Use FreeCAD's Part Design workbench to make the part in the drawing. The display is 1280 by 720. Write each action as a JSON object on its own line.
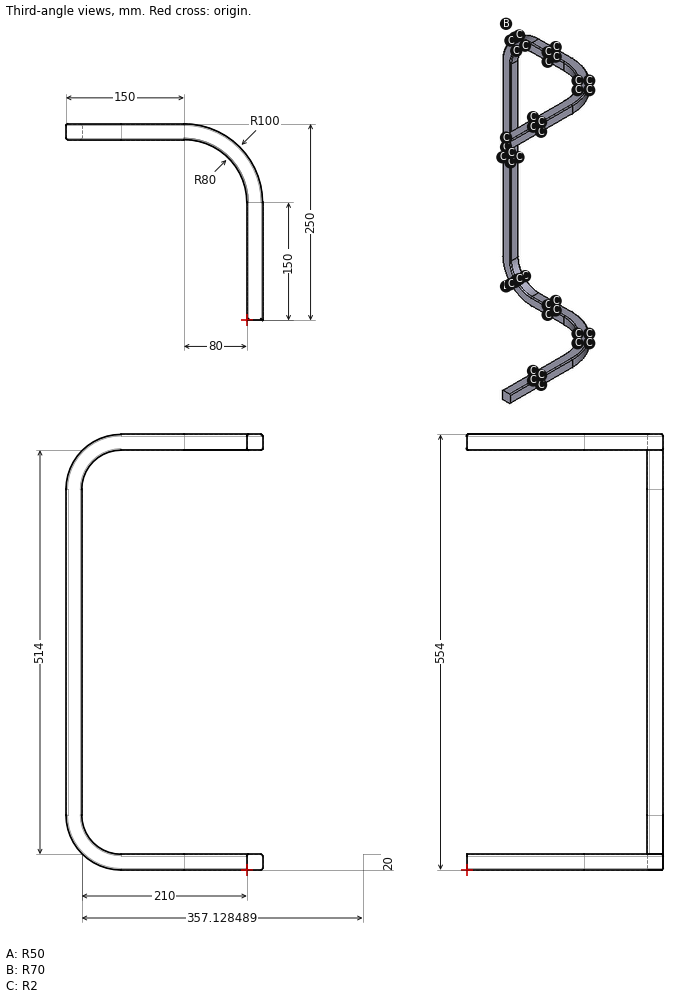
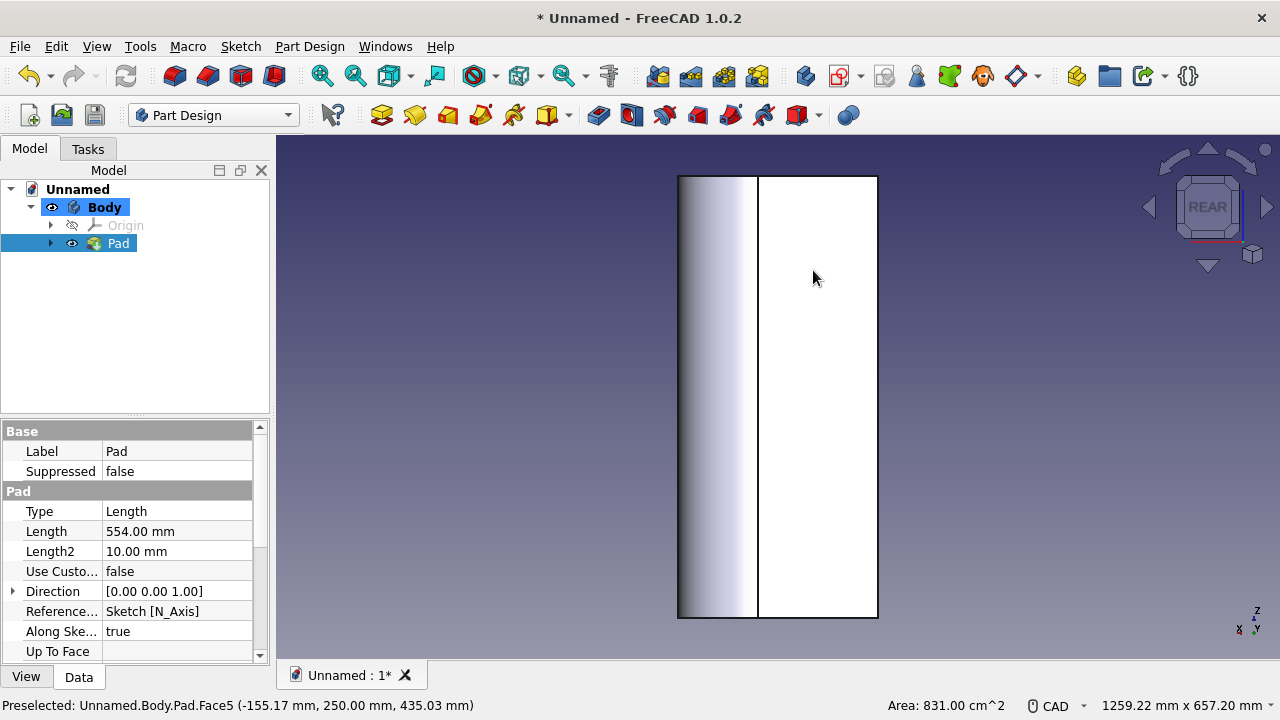
{"action": "left_click", "coordinate": [838, 76]}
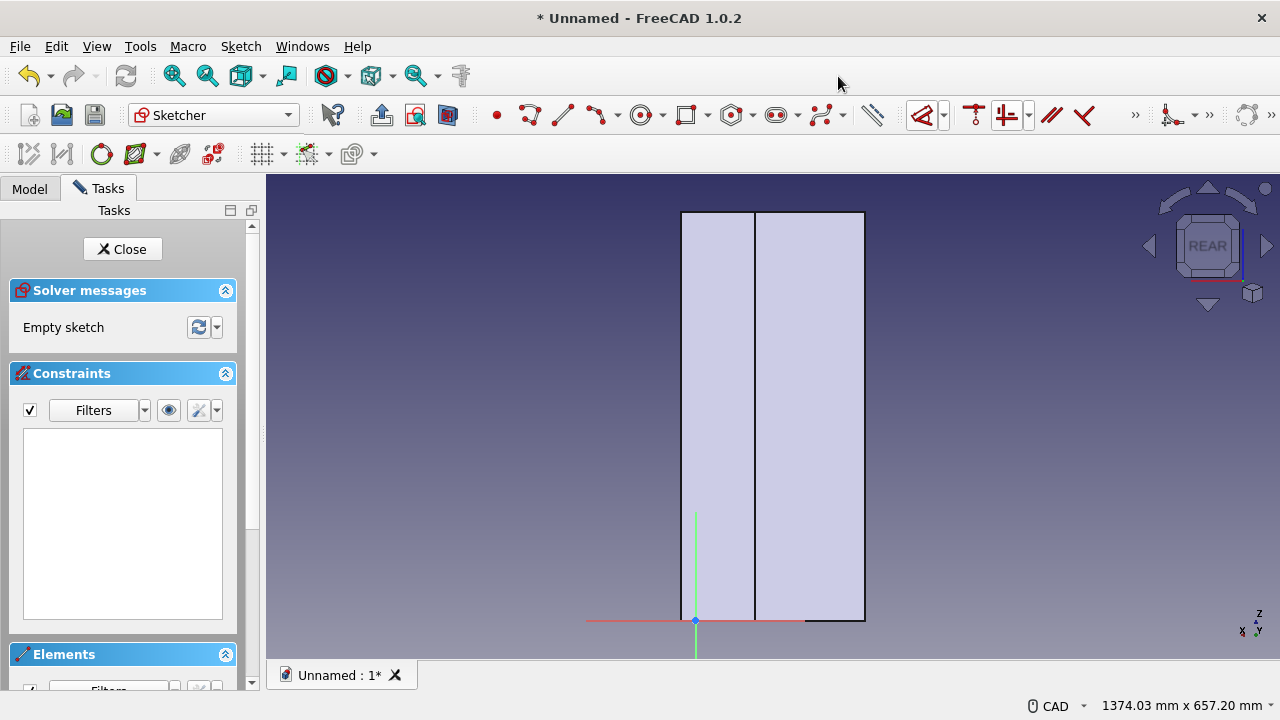
{"action": "scroll", "coordinate": [640, 383], "scroll_direction": "down", "scroll_amount": 1}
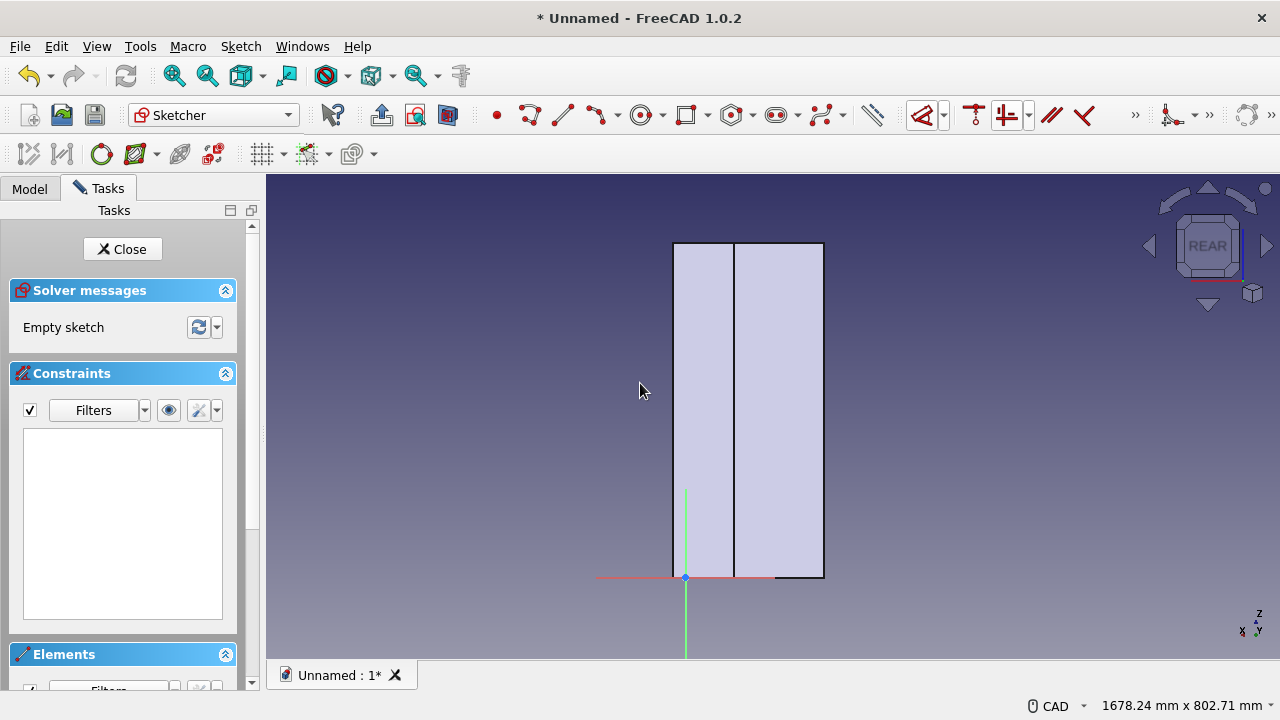
{"action": "left_click", "coordinate": [686, 116]}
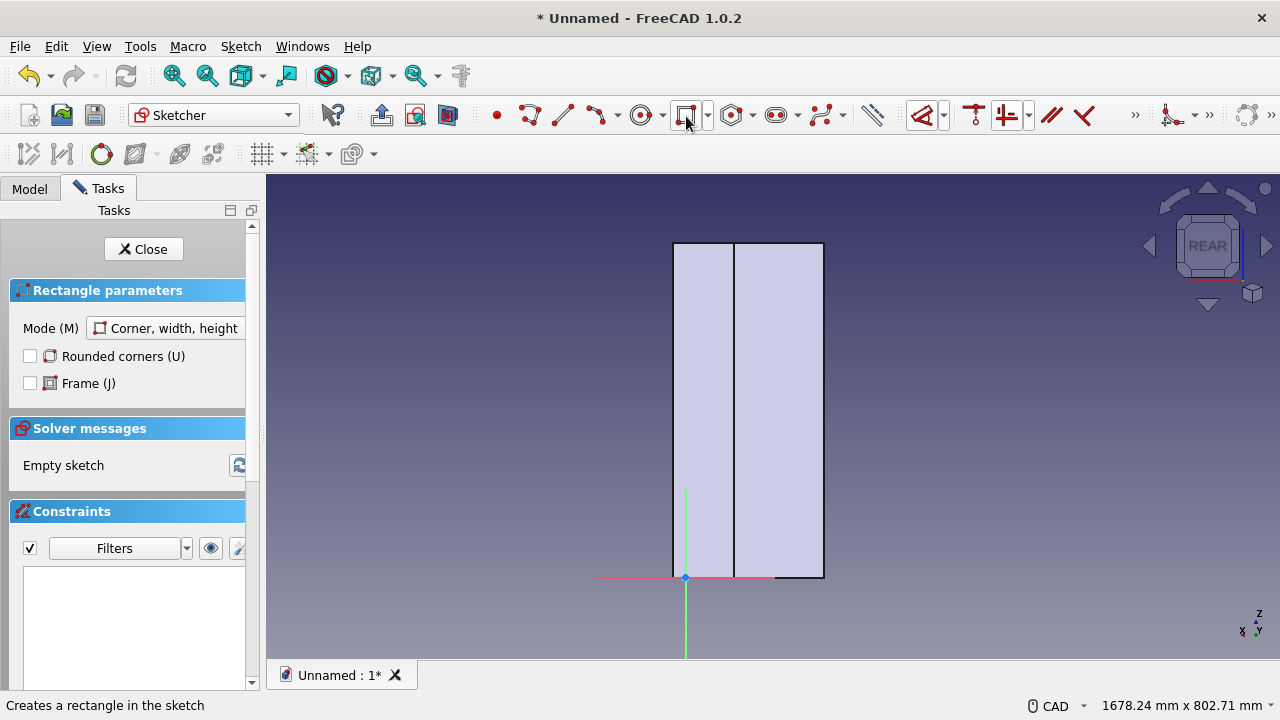
{"action": "left_click", "coordinate": [597, 255]}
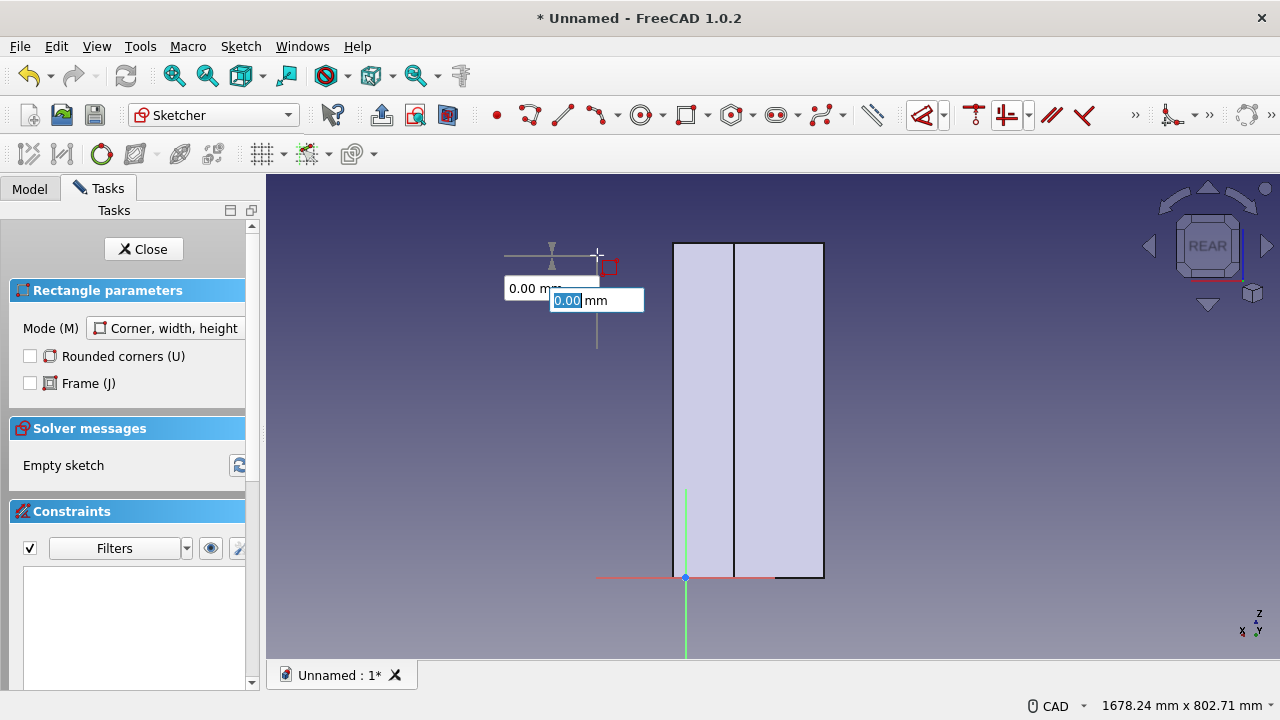
{"action": "scroll", "coordinate": [812, 566], "scroll_direction": "up", "scroll_amount": 2}
{"action": "mouse_move", "coordinate": [812, 565]}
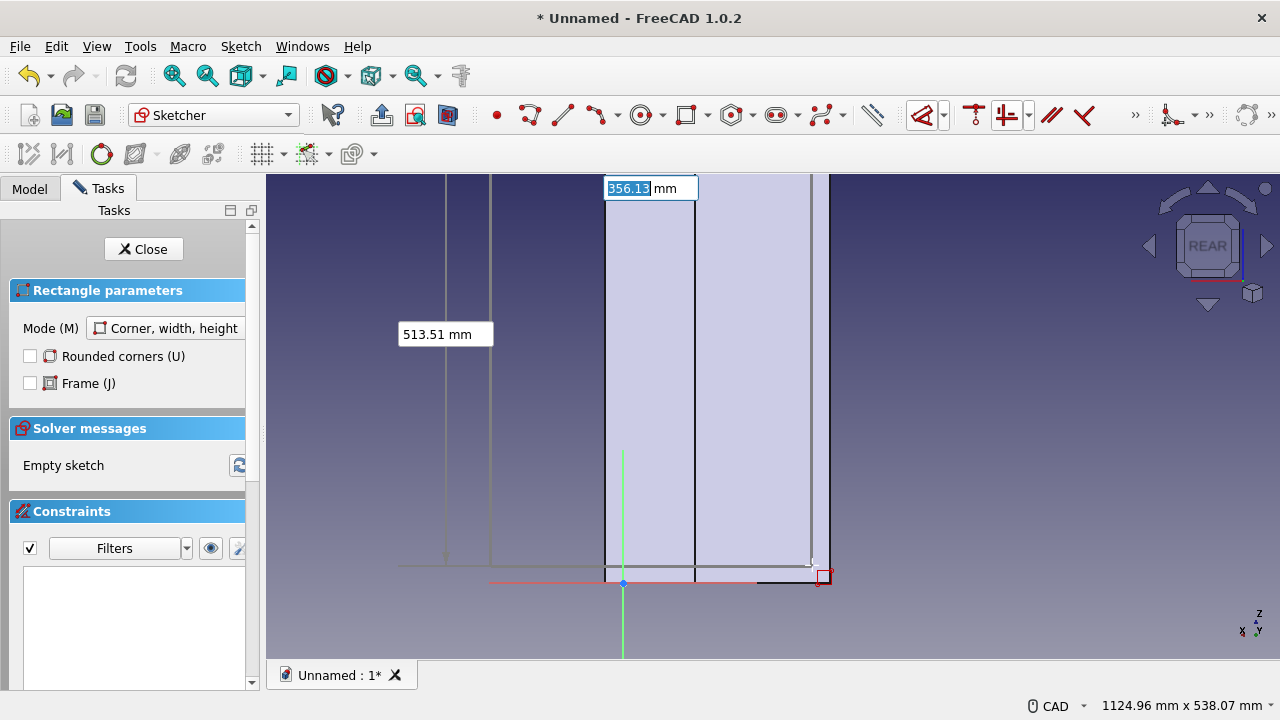
{"action": "type", "text": "357.128489"}
{"action": "key", "text": "Tab"}
{"action": "type", "text": "514"}
{"action": "key", "text": "Return"}
{"action": "key", "text": "Escape"}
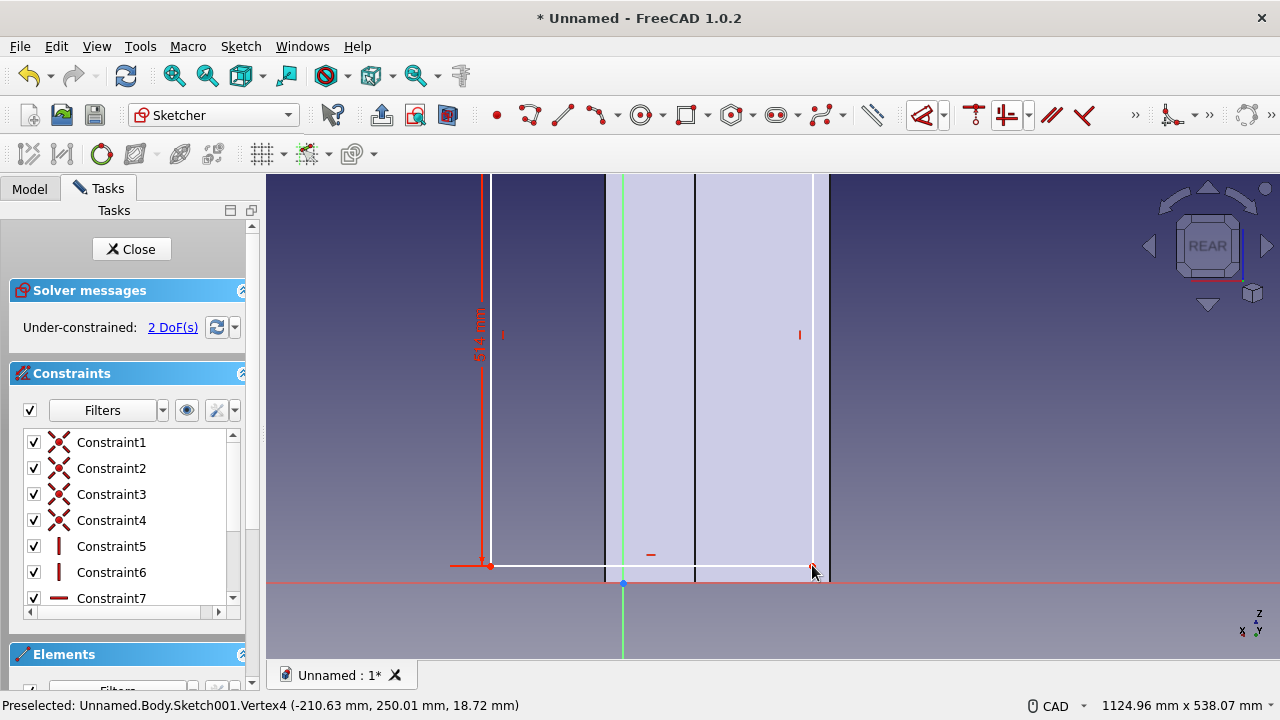
{"action": "scroll", "coordinate": [491, 566], "scroll_direction": "up", "scroll_amount": 4}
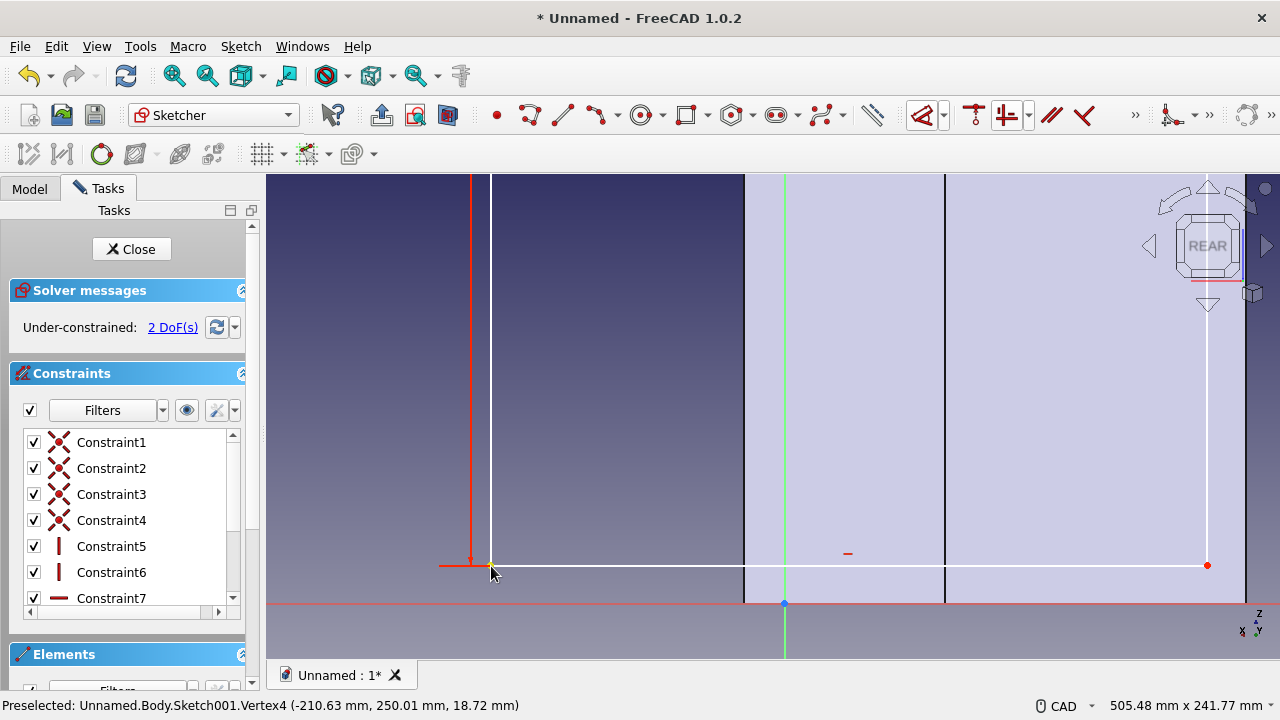
{"action": "left_click", "coordinate": [491, 566]}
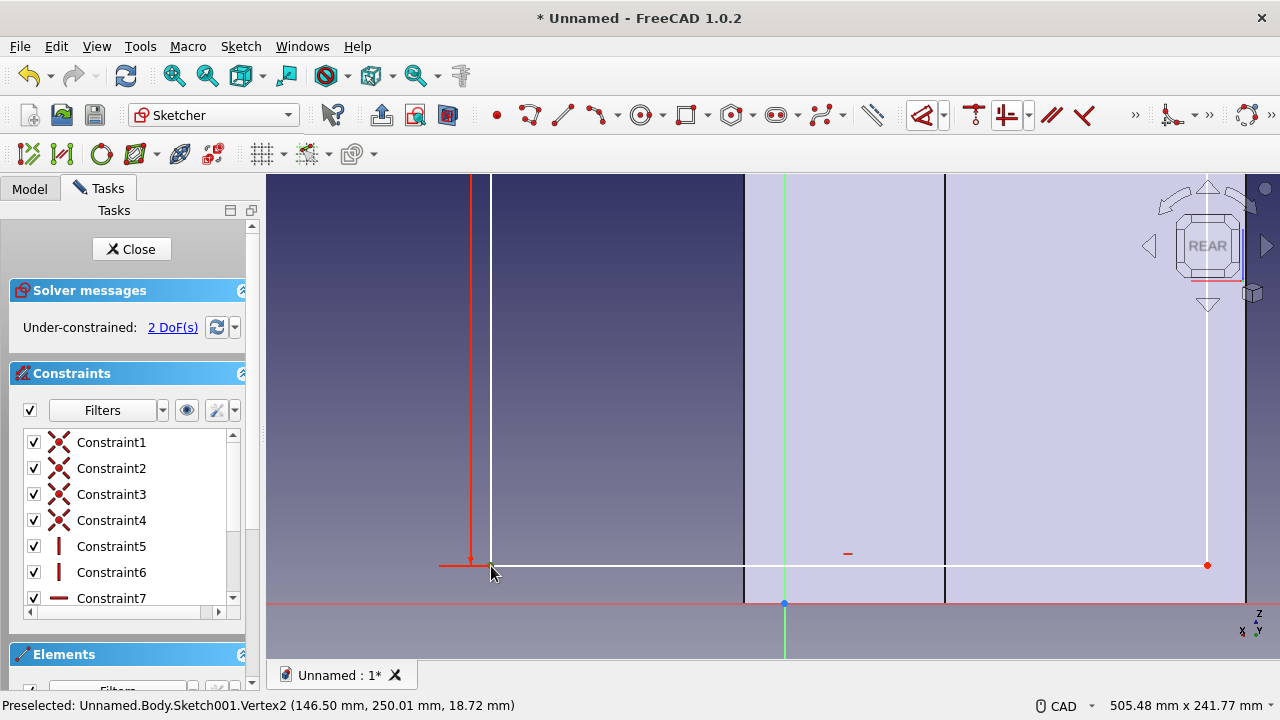
{"action": "key", "text": "i"}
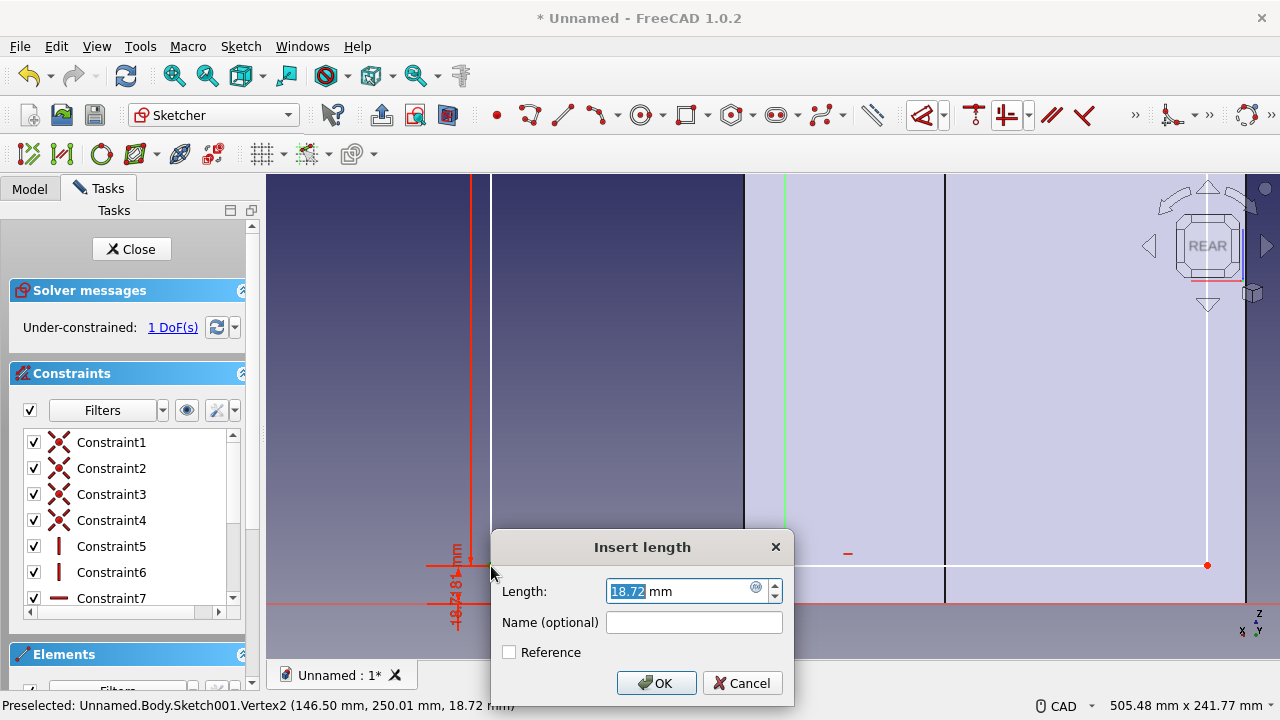
{"action": "type", "text": "20"}
{"action": "key", "text": "Return"}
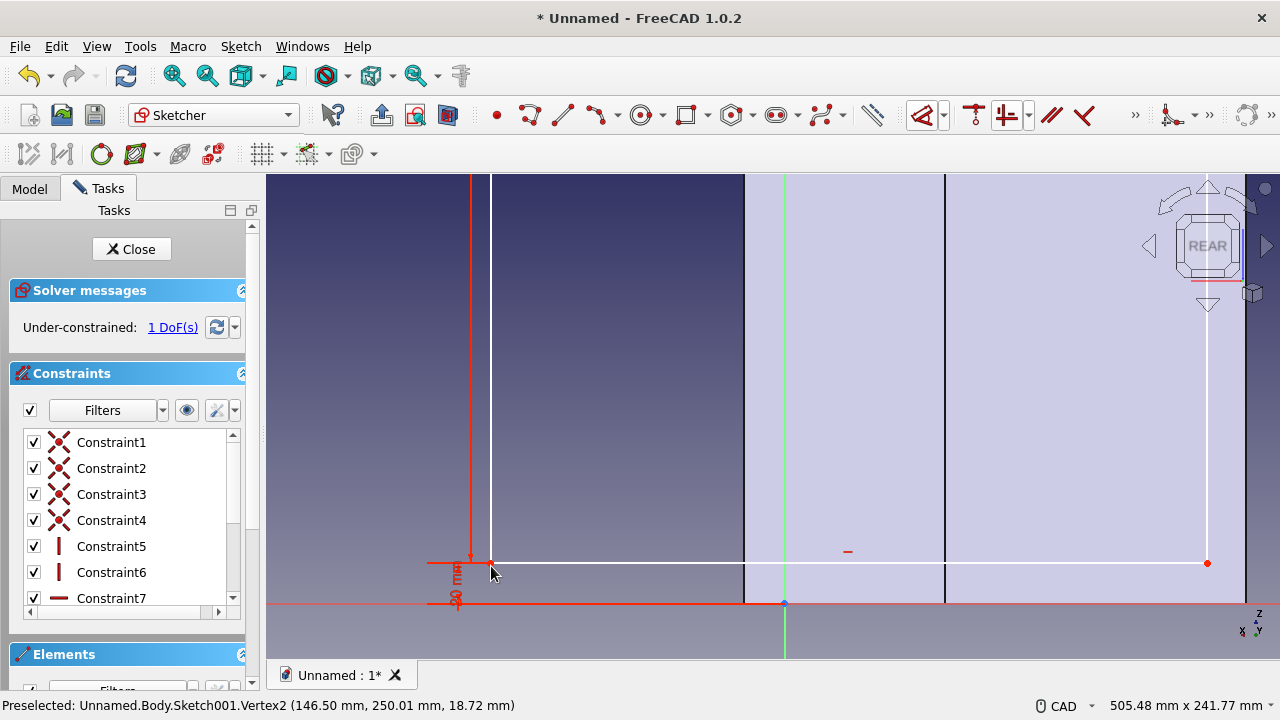
{"action": "scroll", "coordinate": [643, 567], "scroll_direction": "down", "scroll_amount": 6}